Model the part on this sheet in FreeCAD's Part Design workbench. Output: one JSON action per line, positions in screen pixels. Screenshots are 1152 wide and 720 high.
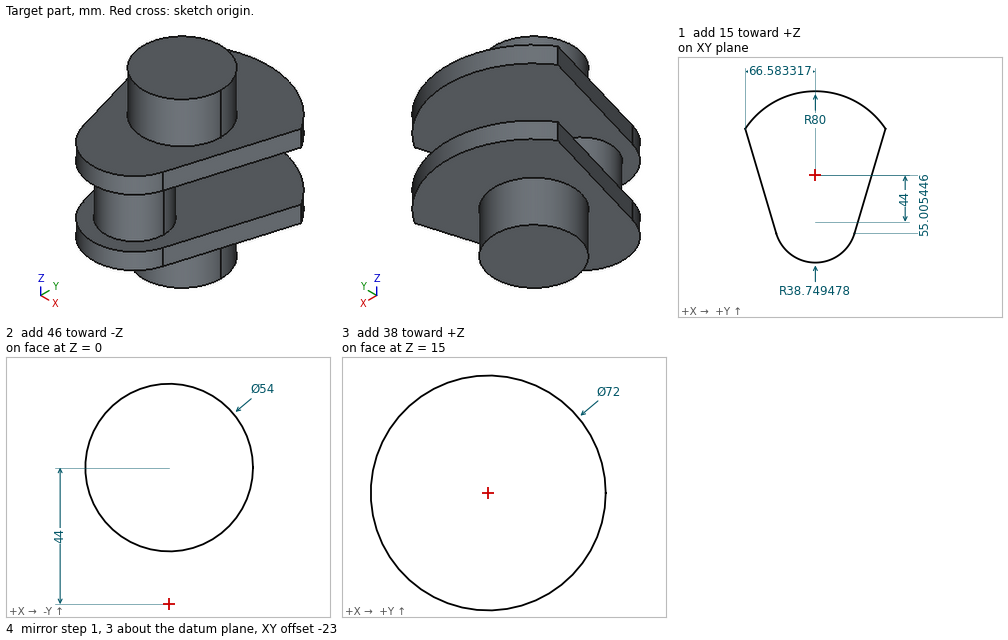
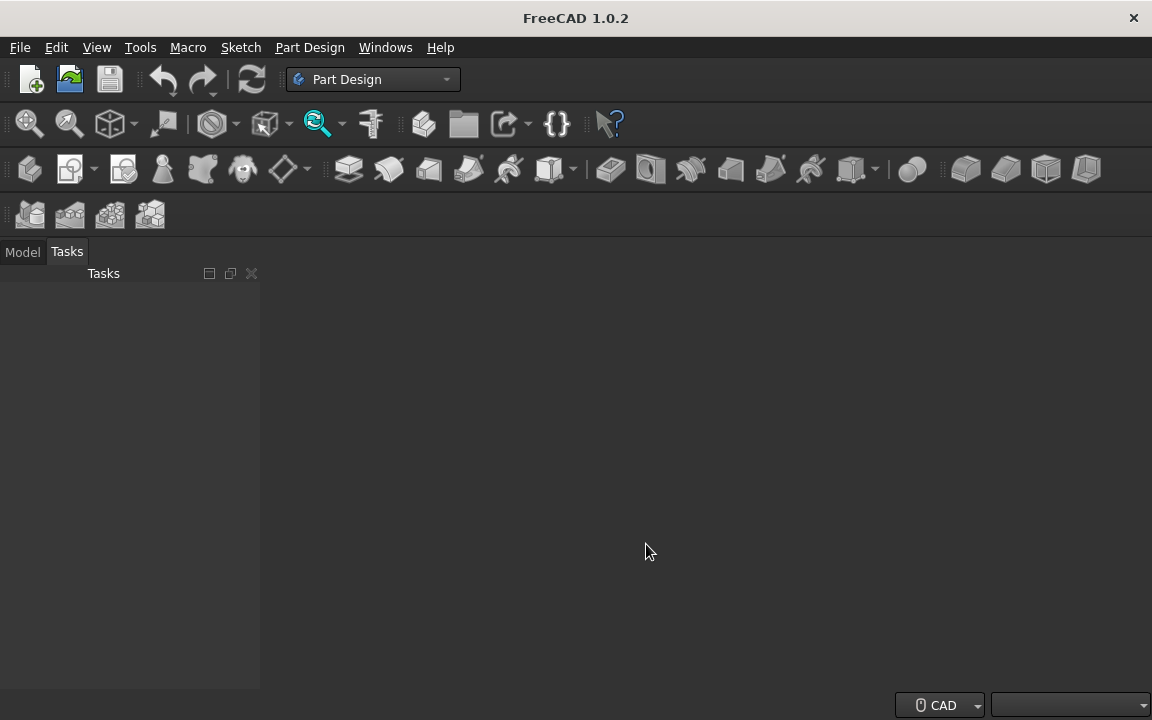
{"action": "left_click", "coordinate": [30, 80]}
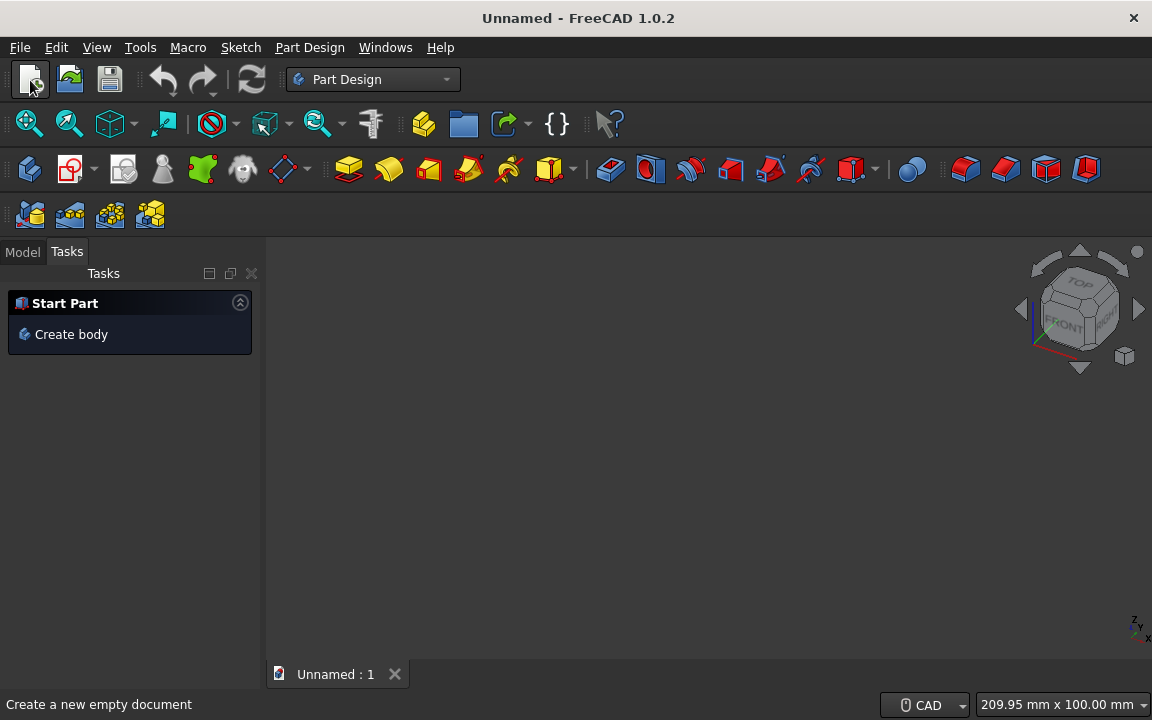
{"action": "left_click", "coordinate": [70, 170]}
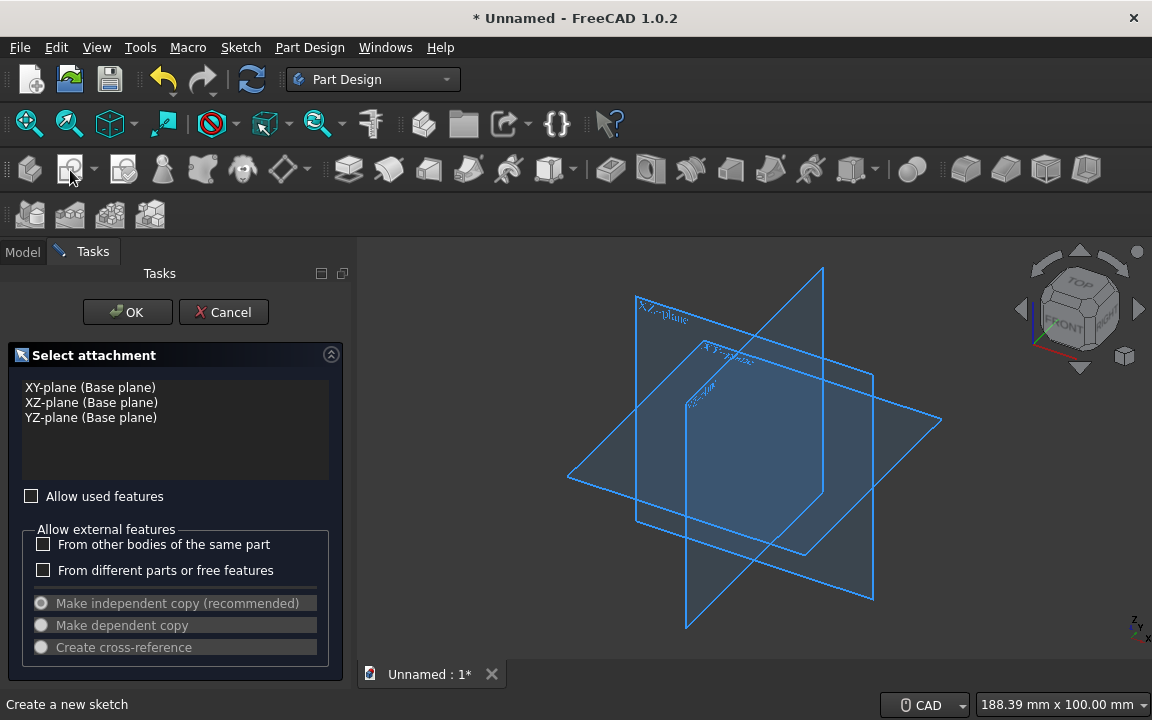
{"action": "left_click", "coordinate": [82, 388]}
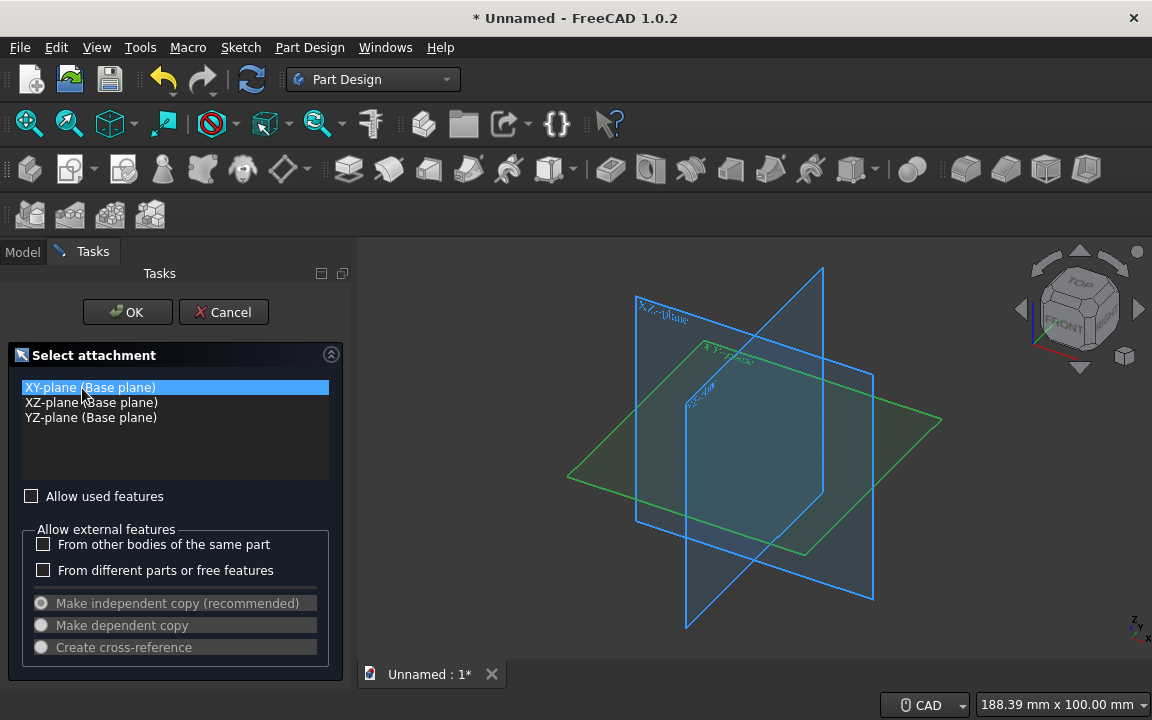
{"action": "left_click", "coordinate": [128, 312]}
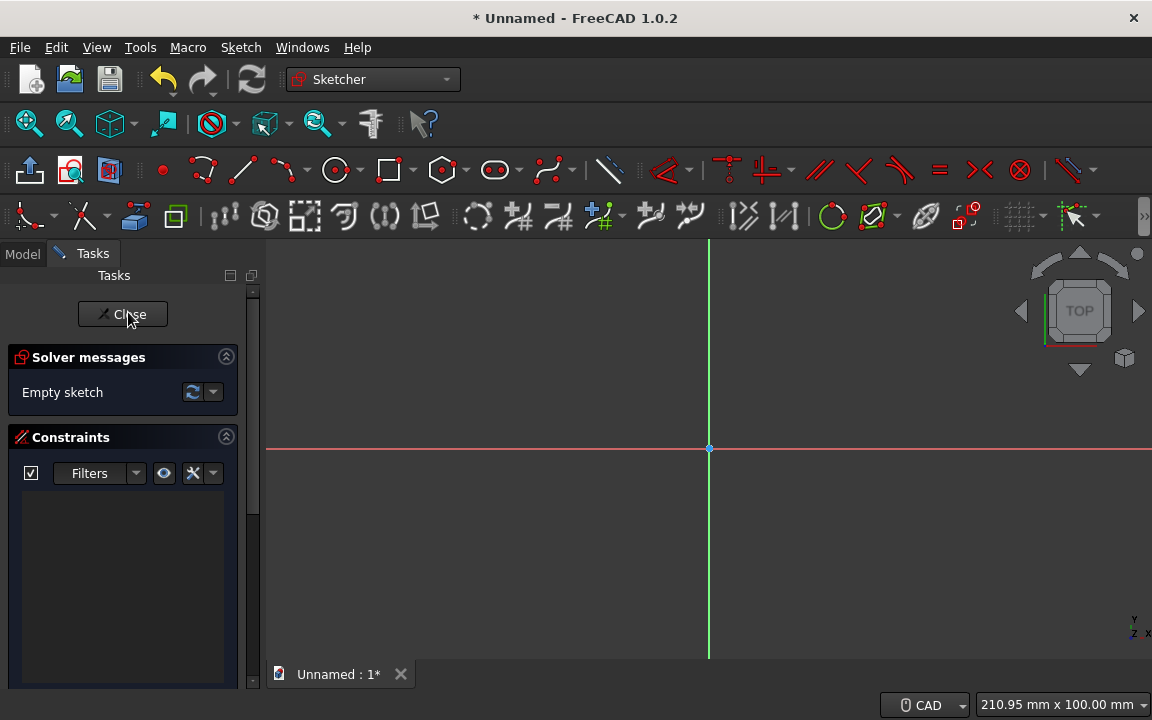
{"action": "scroll", "coordinate": [601, 446], "scroll_direction": "down", "scroll_amount": 5}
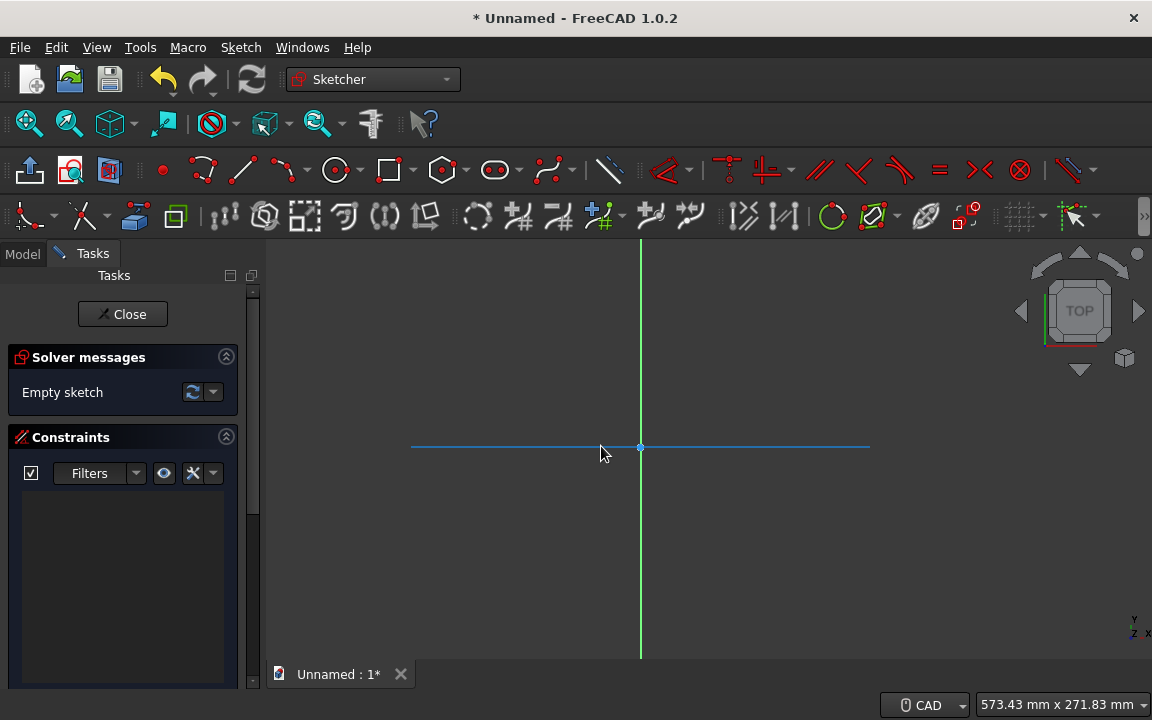
{"action": "left_click", "coordinate": [244, 170]}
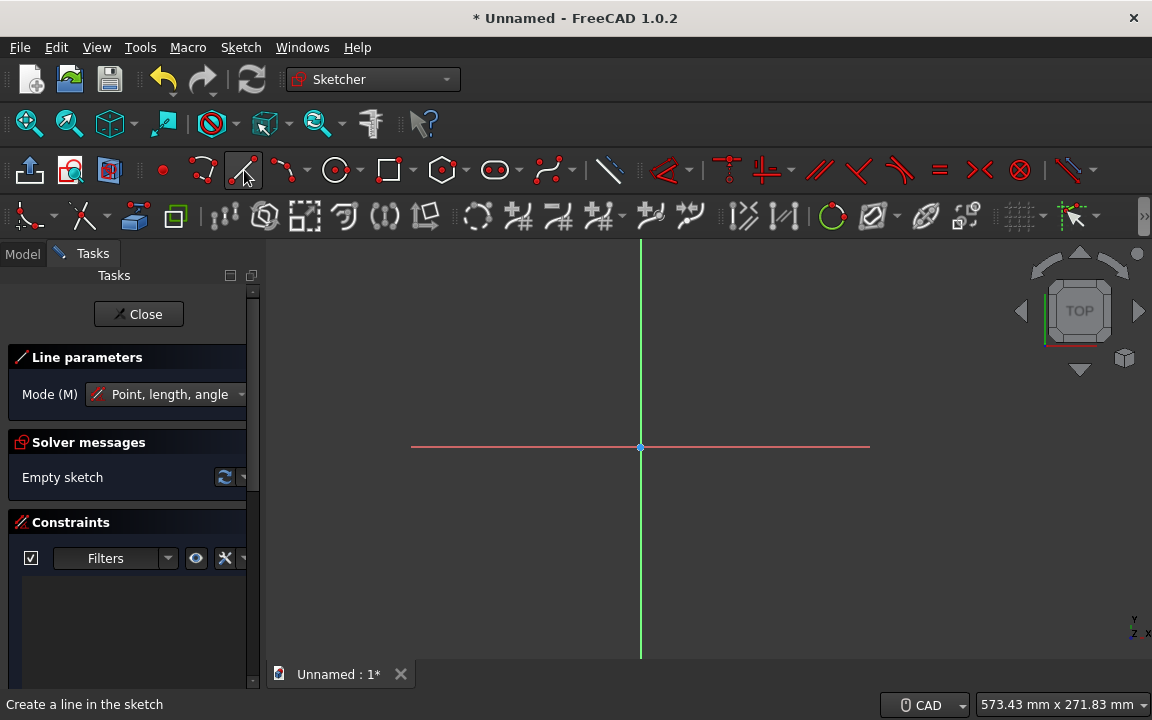
{"action": "left_click", "coordinate": [538, 379]}
{"action": "left_click", "coordinate": [584, 532]}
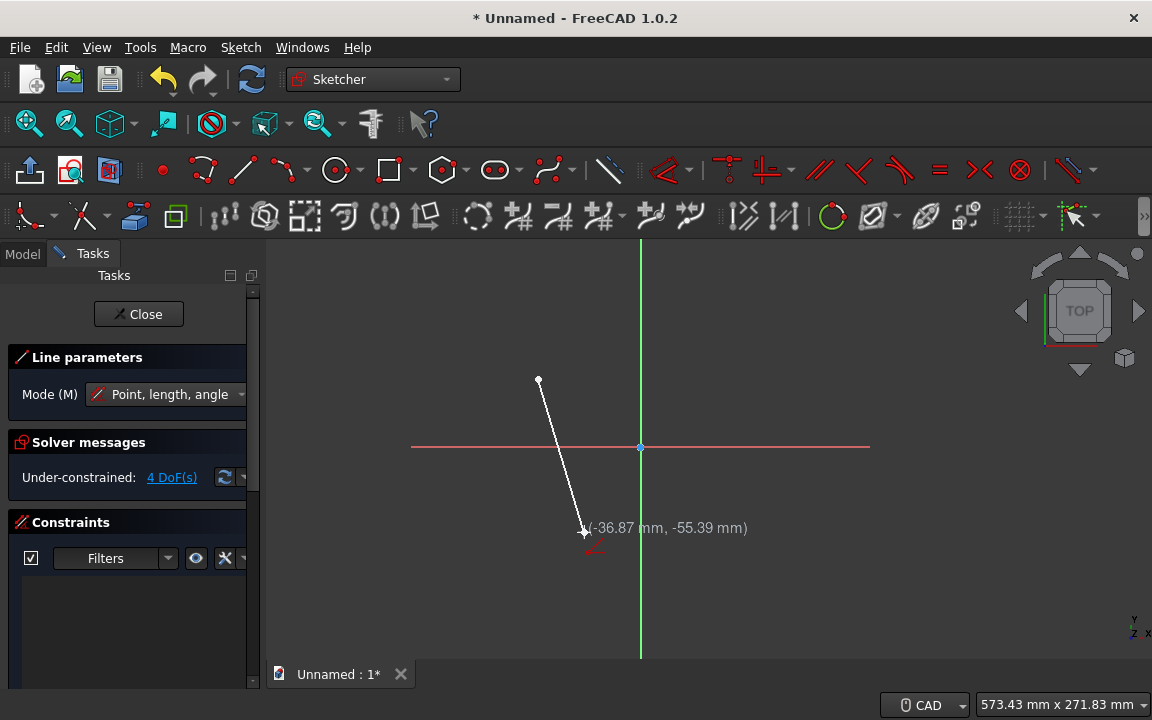
{"action": "left_click", "coordinate": [698, 532]}
{"action": "left_click", "coordinate": [744, 379]}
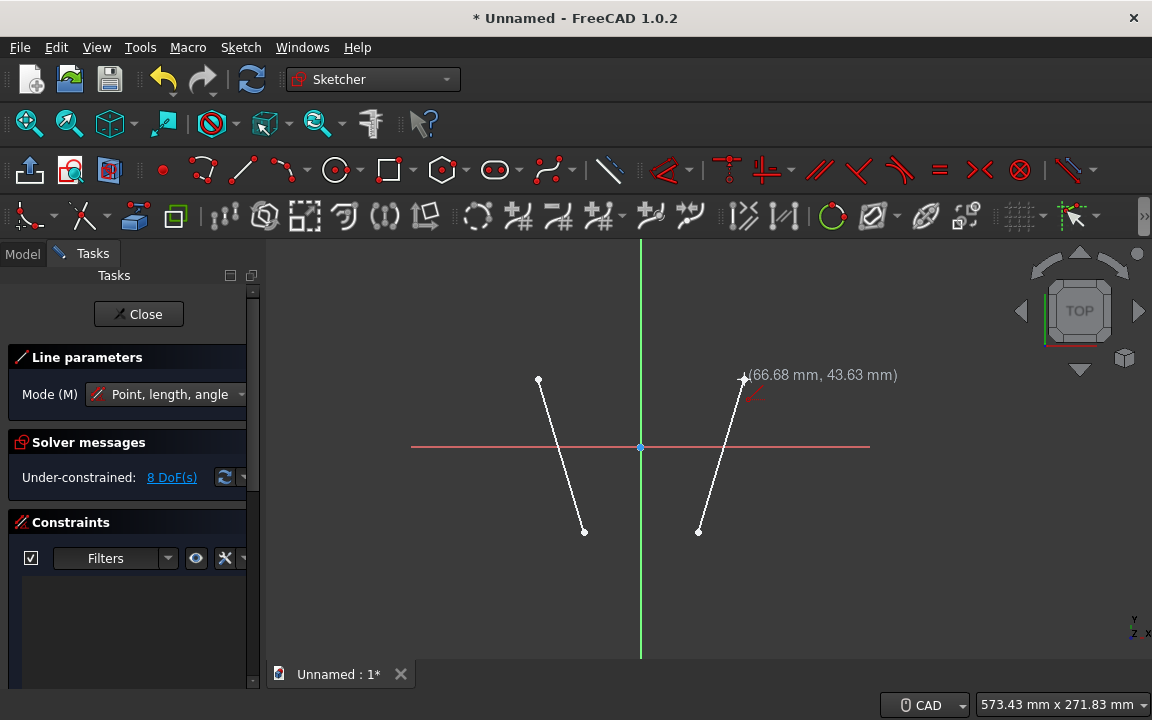
{"action": "left_click", "coordinate": [284, 170]}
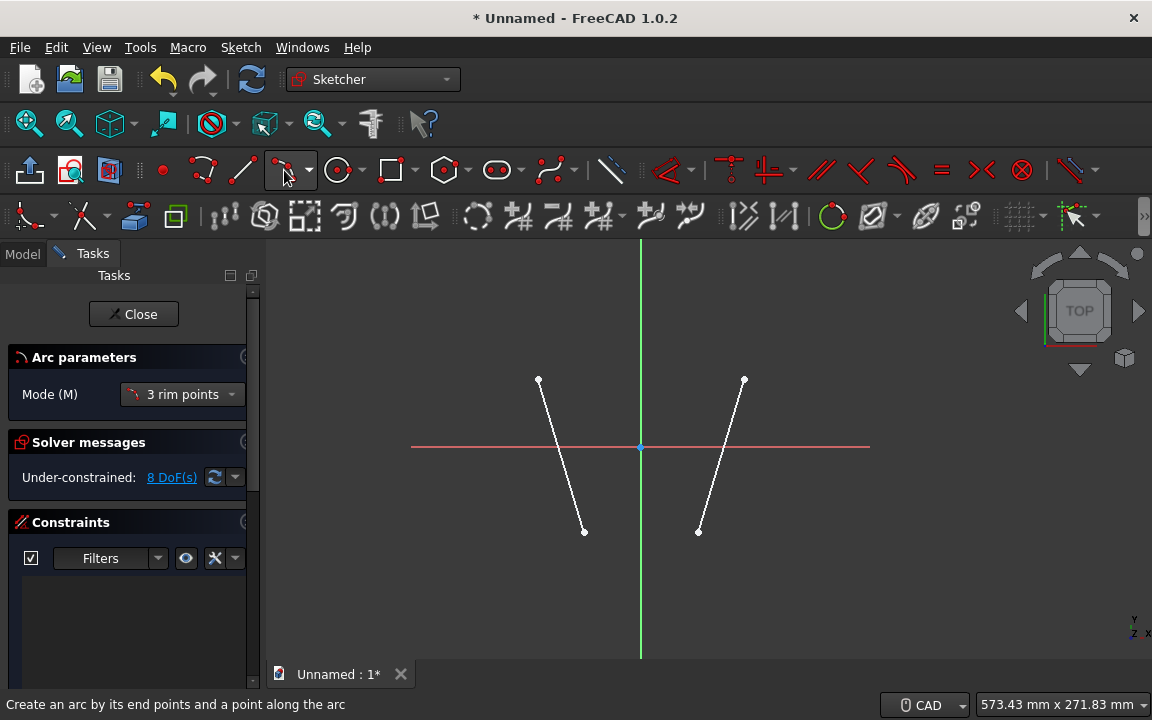
{"action": "left_click", "coordinate": [584, 533]}
{"action": "left_click", "coordinate": [698, 533]}
{"action": "left_click", "coordinate": [626, 573]}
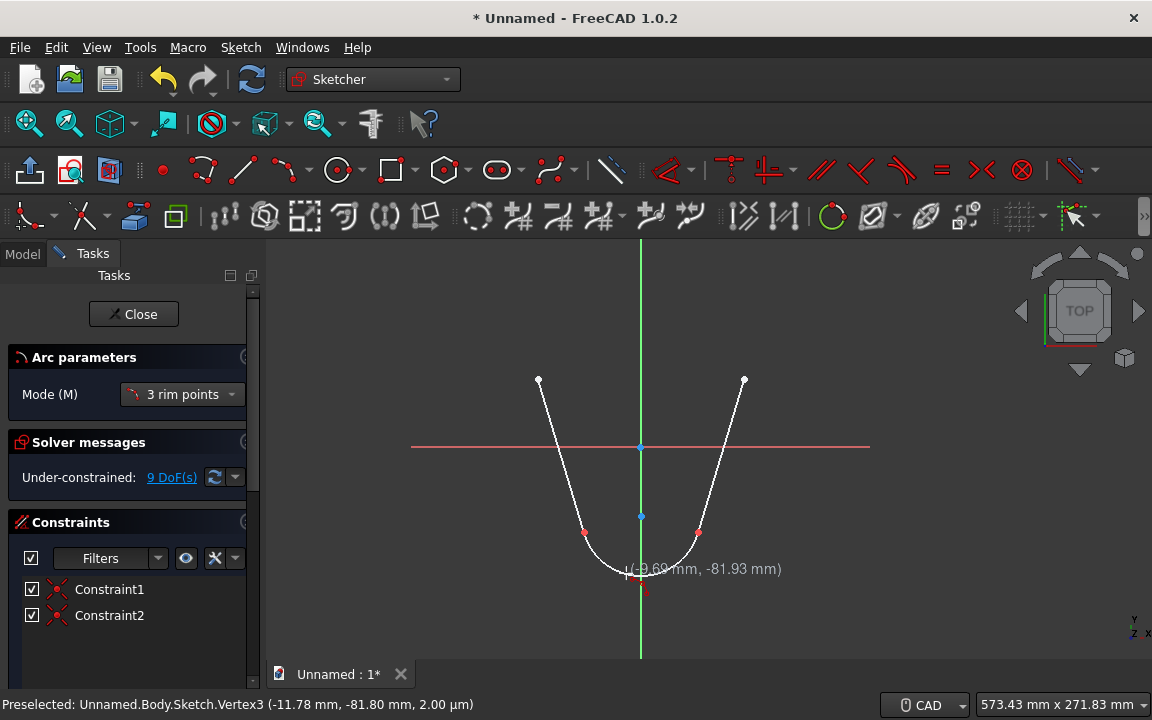
{"action": "left_click", "coordinate": [744, 380]}
{"action": "left_click", "coordinate": [538, 380]}
{"action": "left_click", "coordinate": [665, 326]}
{"action": "key", "text": "Escape"}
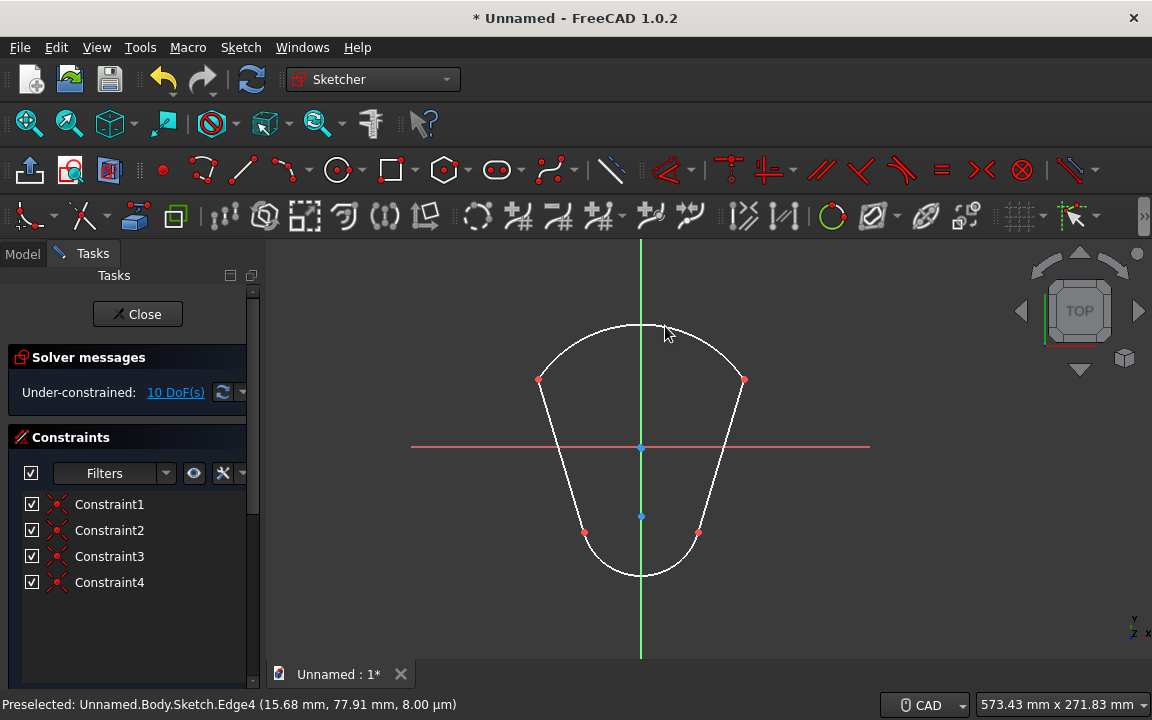
{"action": "left_click", "coordinate": [552, 426]}